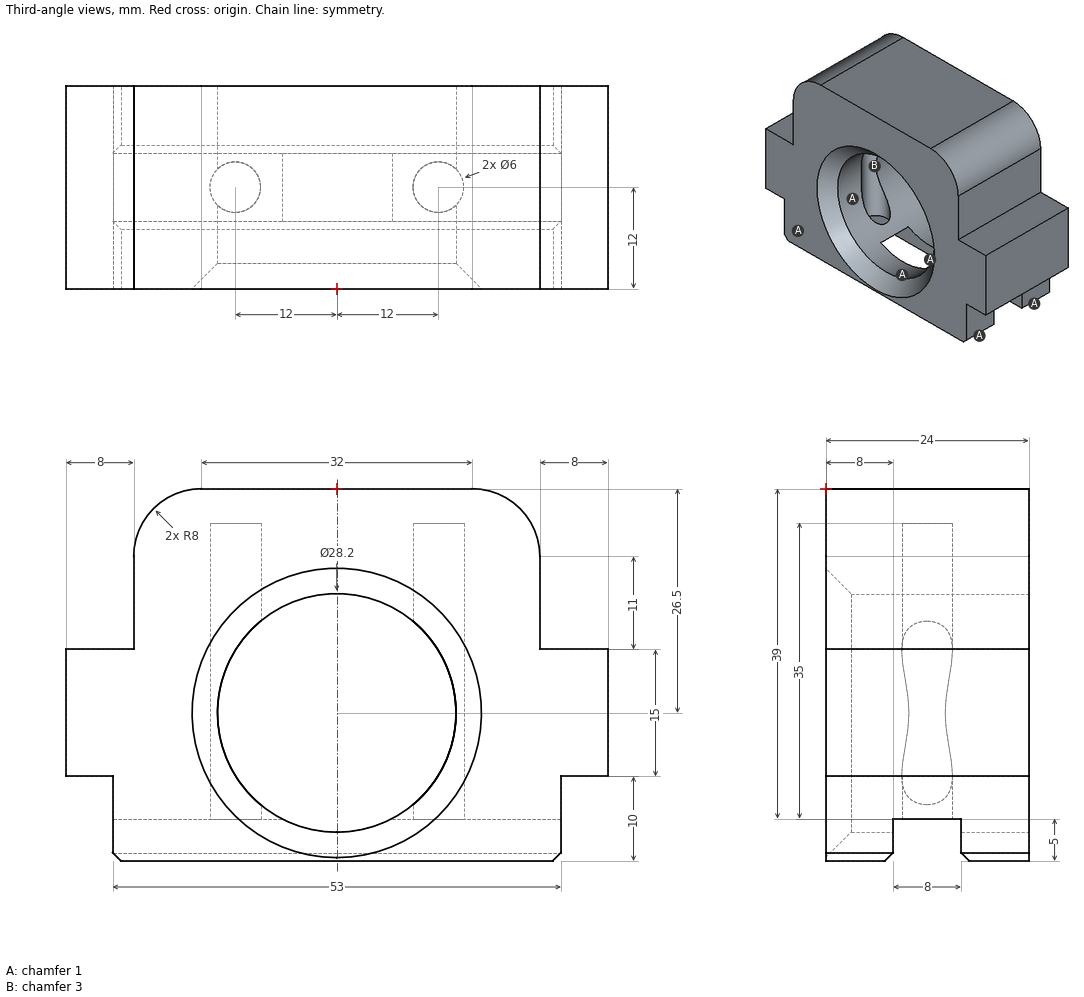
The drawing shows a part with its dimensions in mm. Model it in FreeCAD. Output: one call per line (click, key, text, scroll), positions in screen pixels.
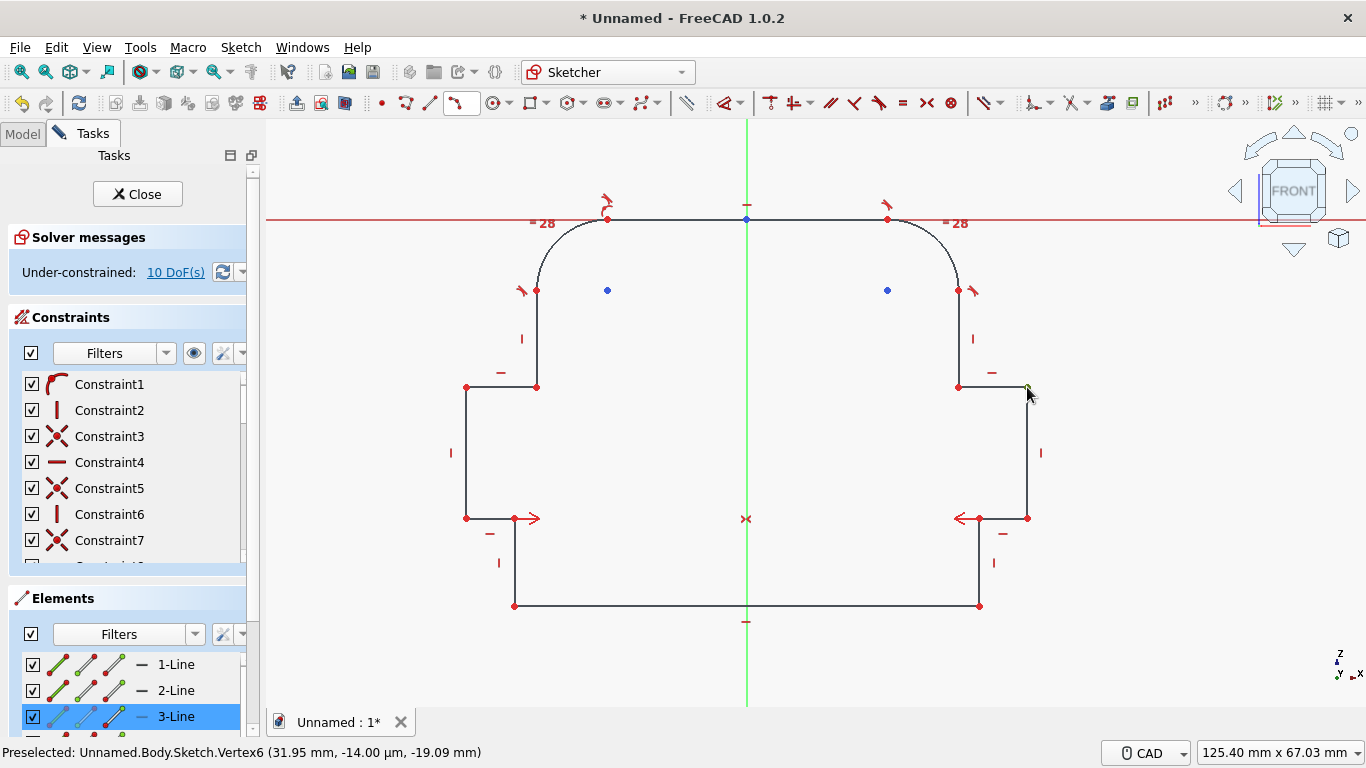
click(466, 387)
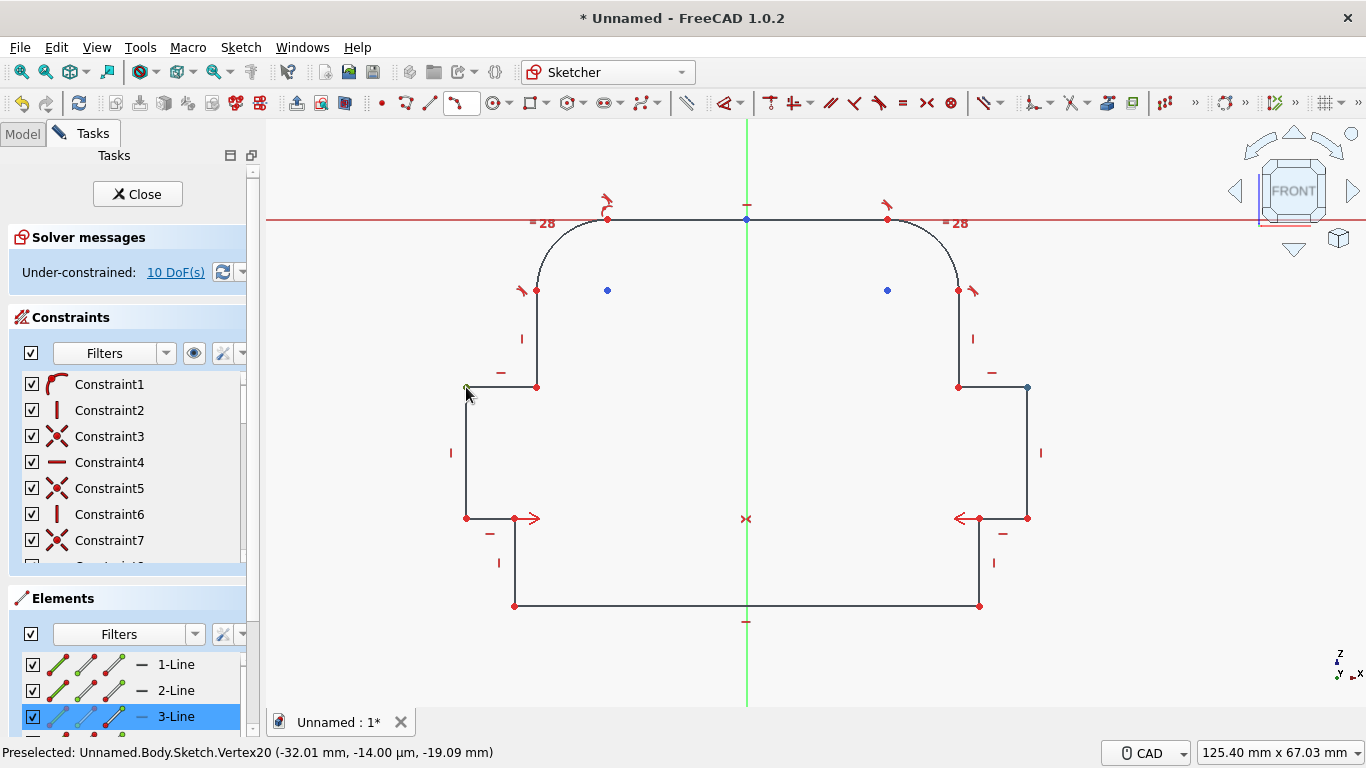
click(747, 641)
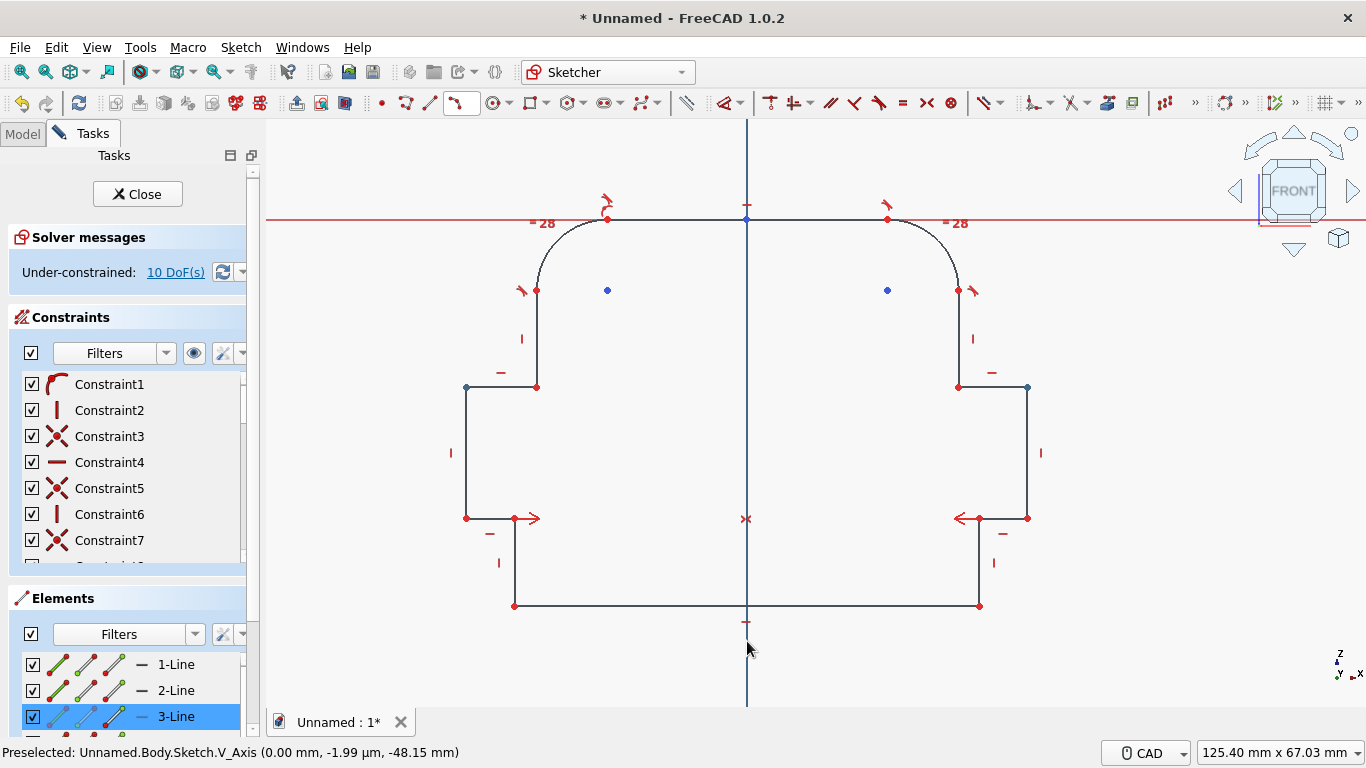
click(928, 104)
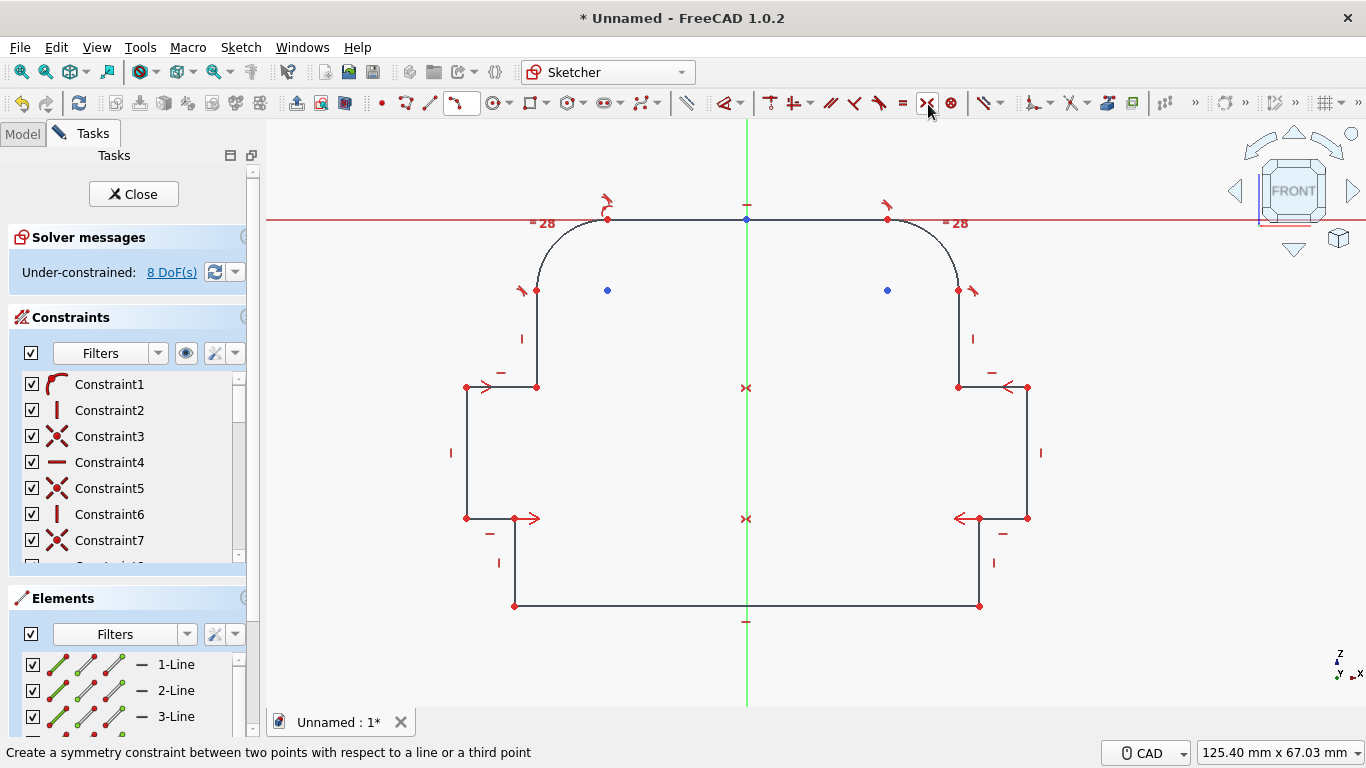
click(951, 258)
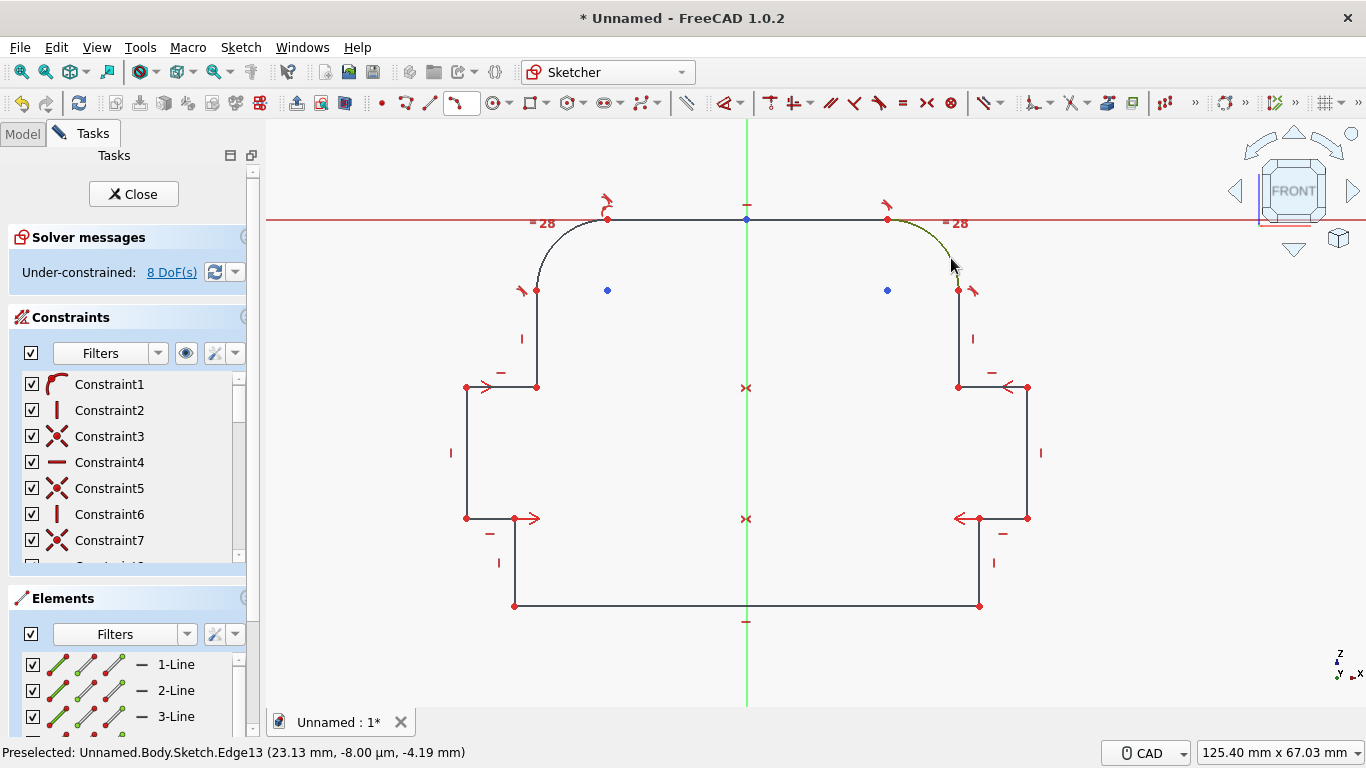
key(k)
key(r)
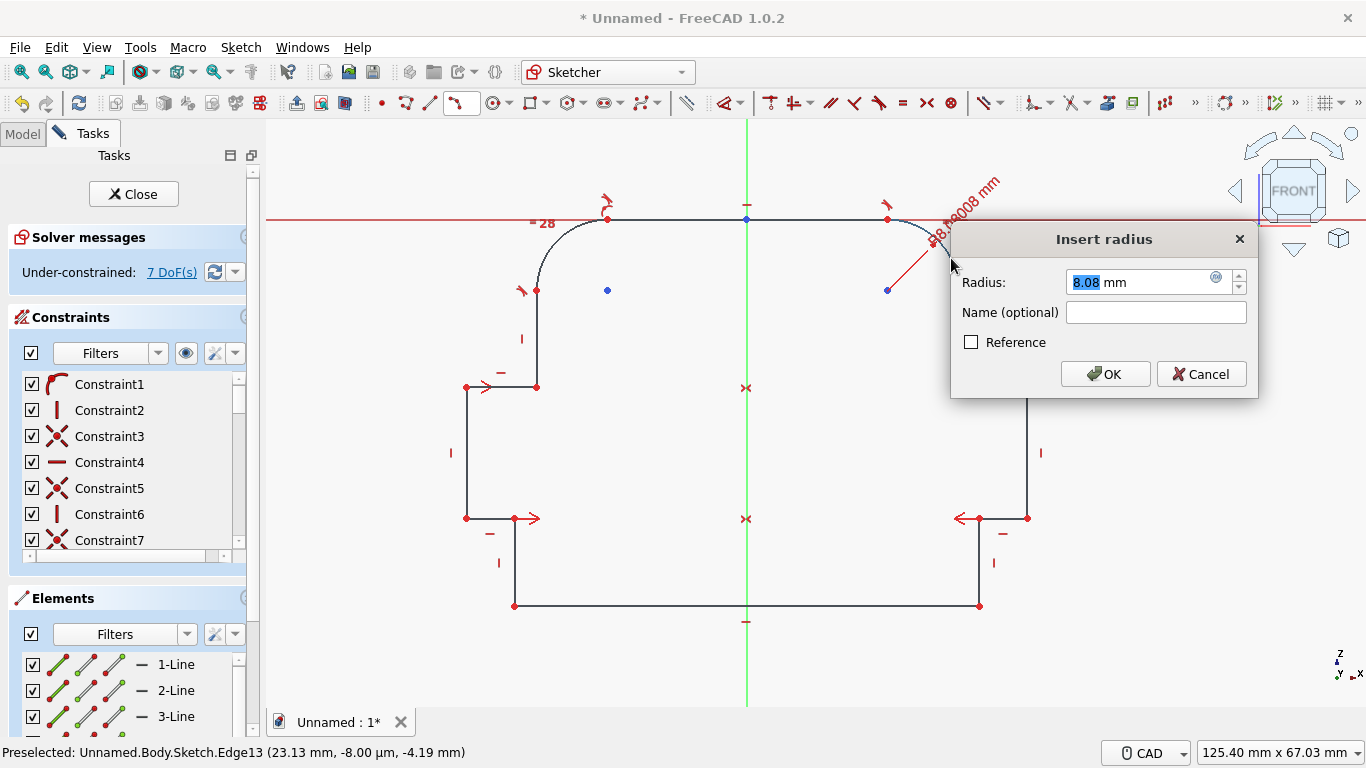
text(8)
key(Return)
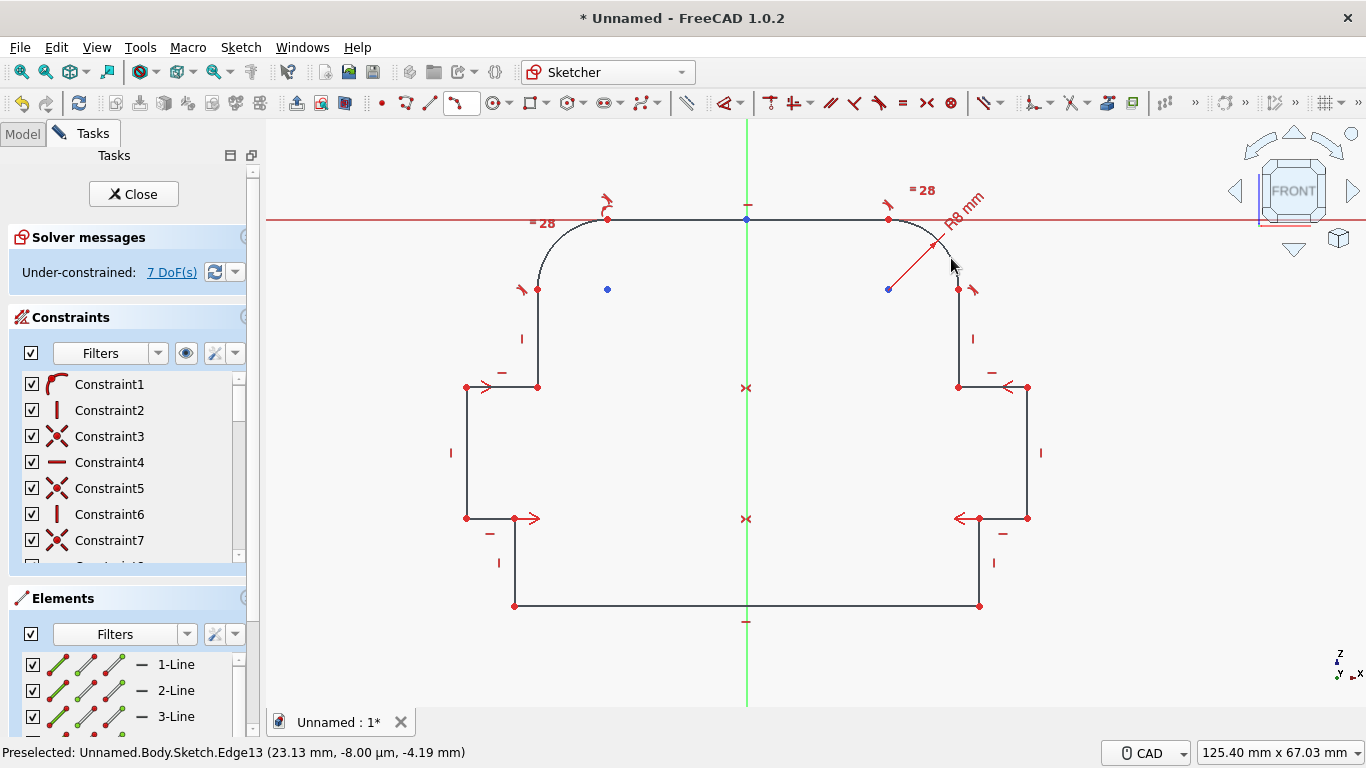
click(979, 387)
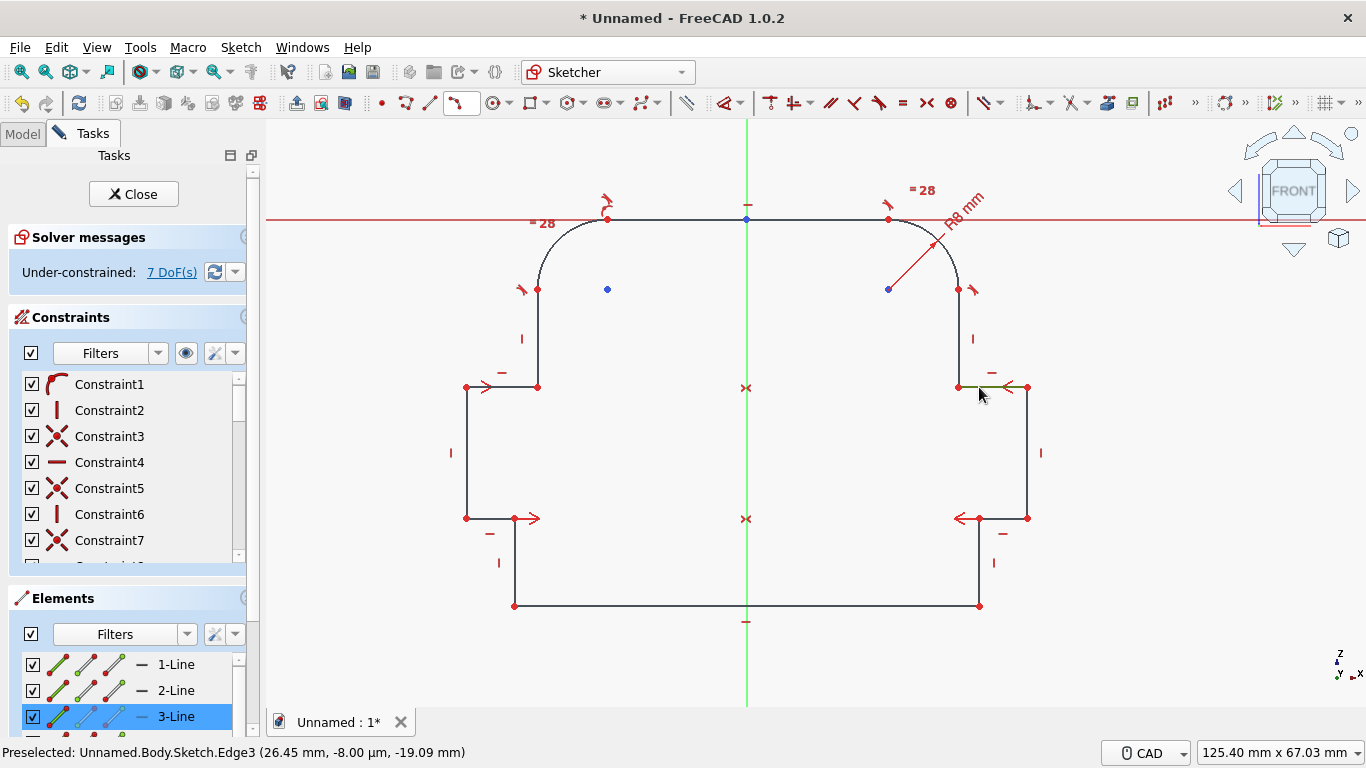
click(742, 104)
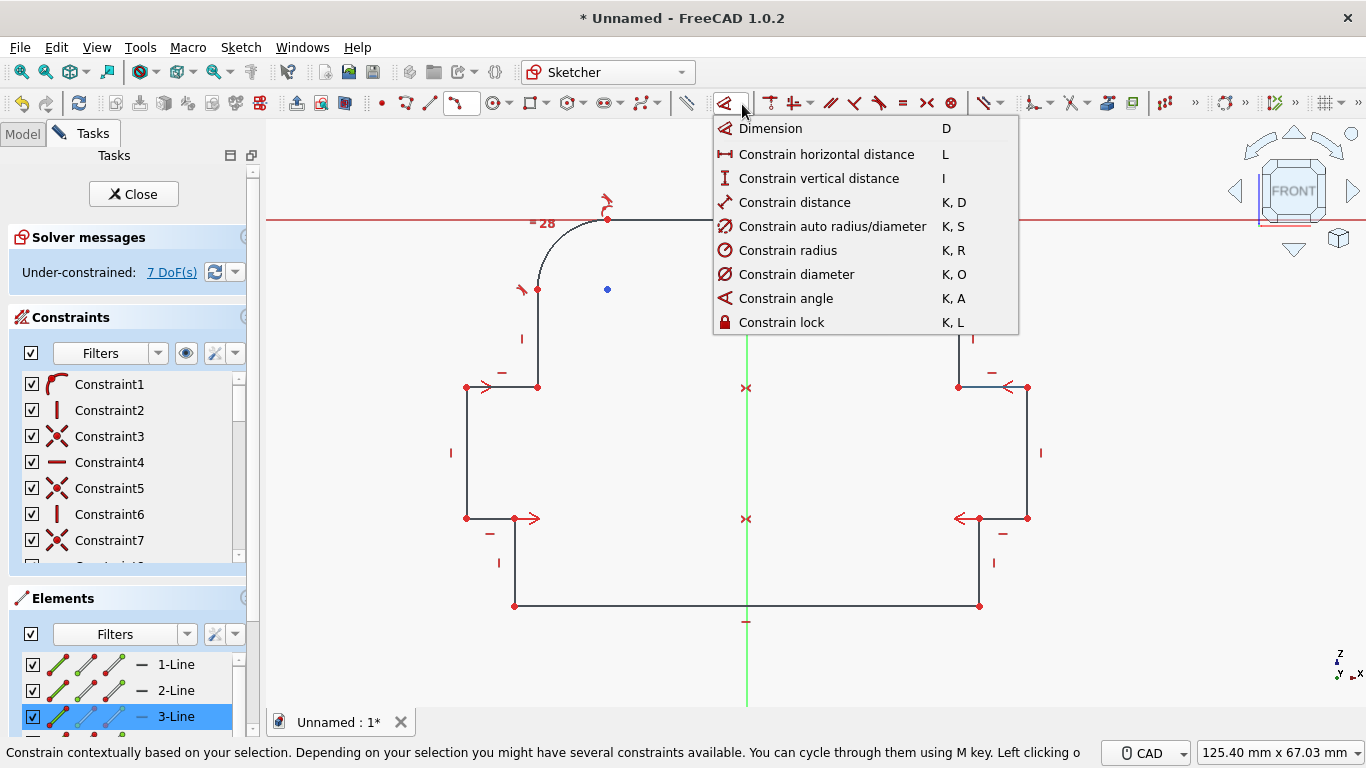
click(866, 154)